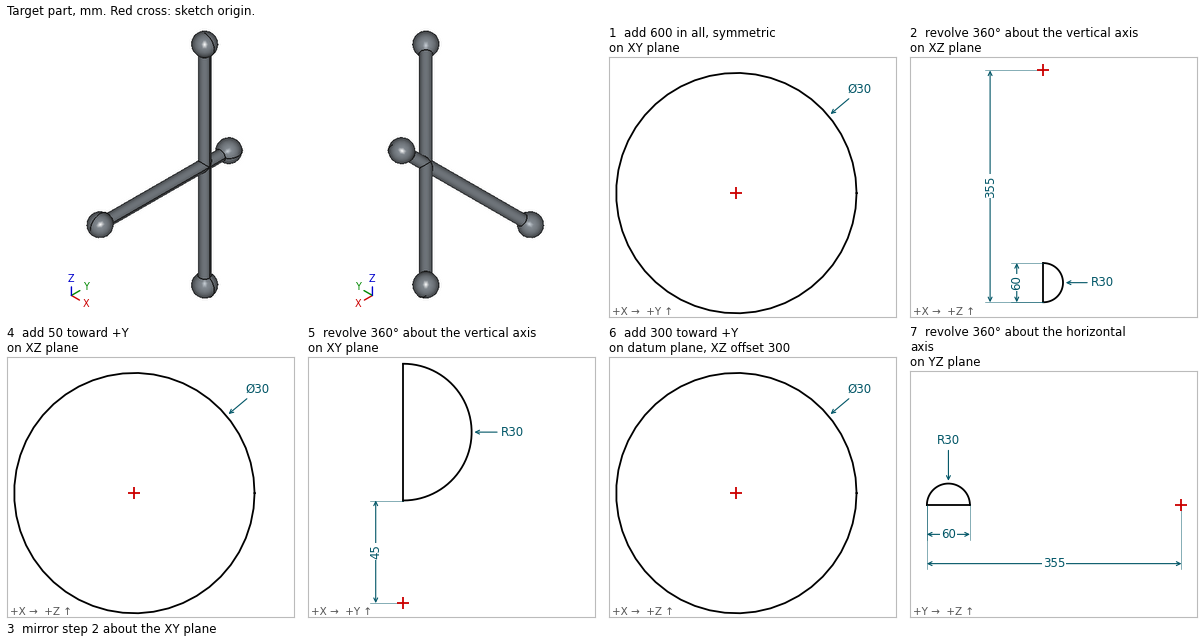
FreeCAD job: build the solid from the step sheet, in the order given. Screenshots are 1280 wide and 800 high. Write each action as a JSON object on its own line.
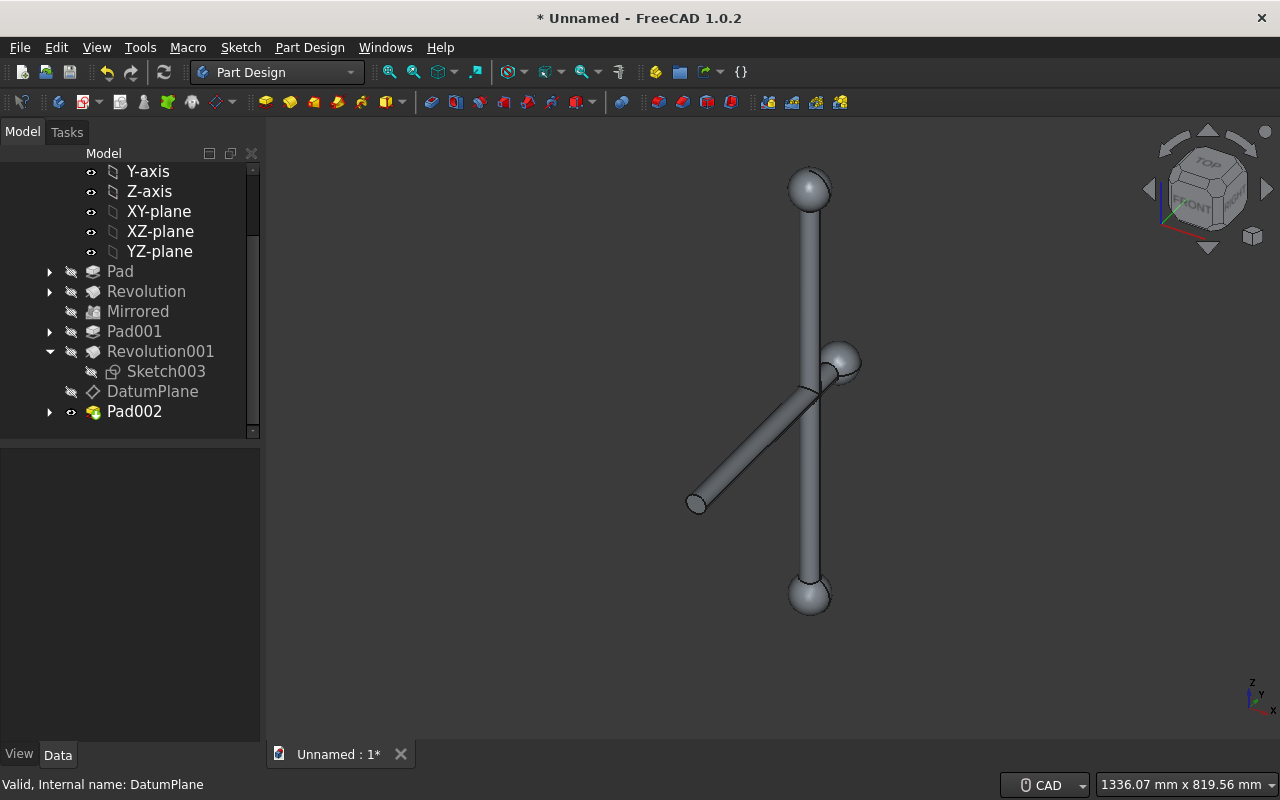
{"action": "left_click", "coordinate": [84, 102]}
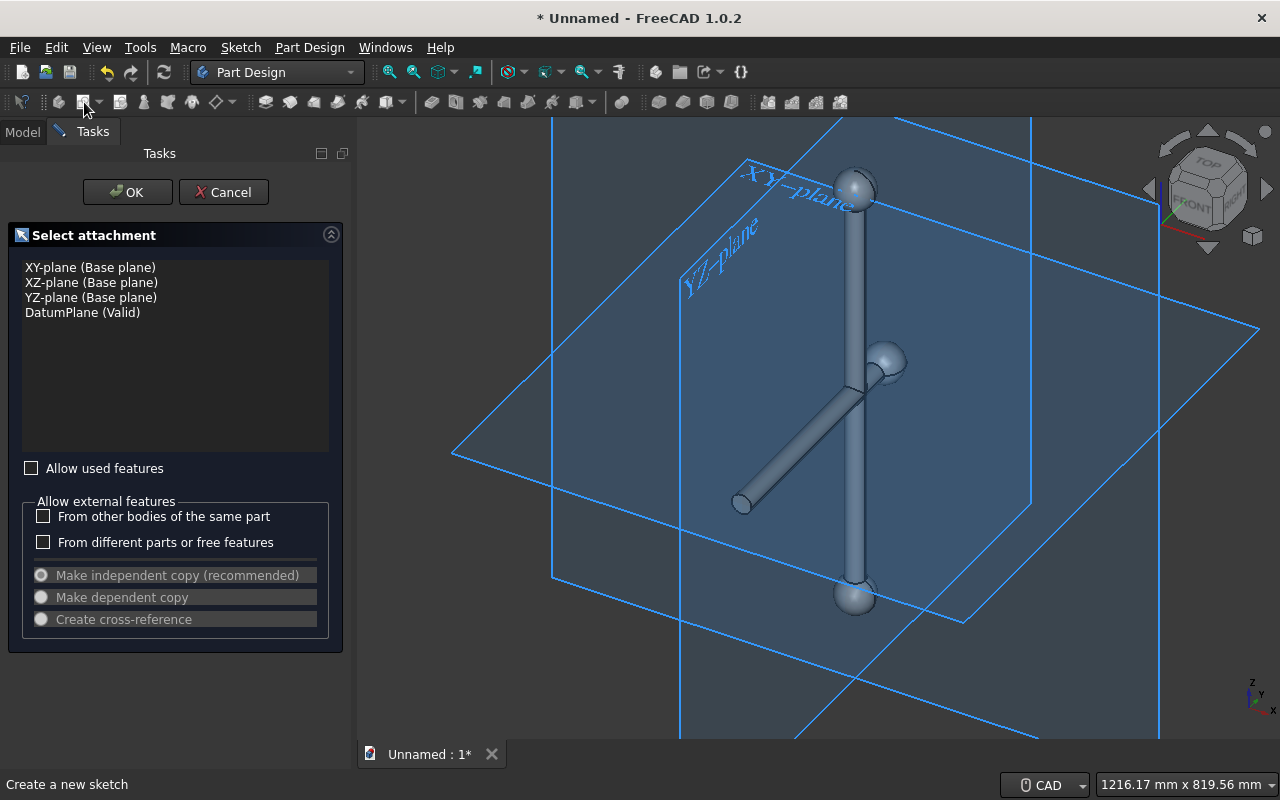
{"action": "left_click", "coordinate": [82, 298]}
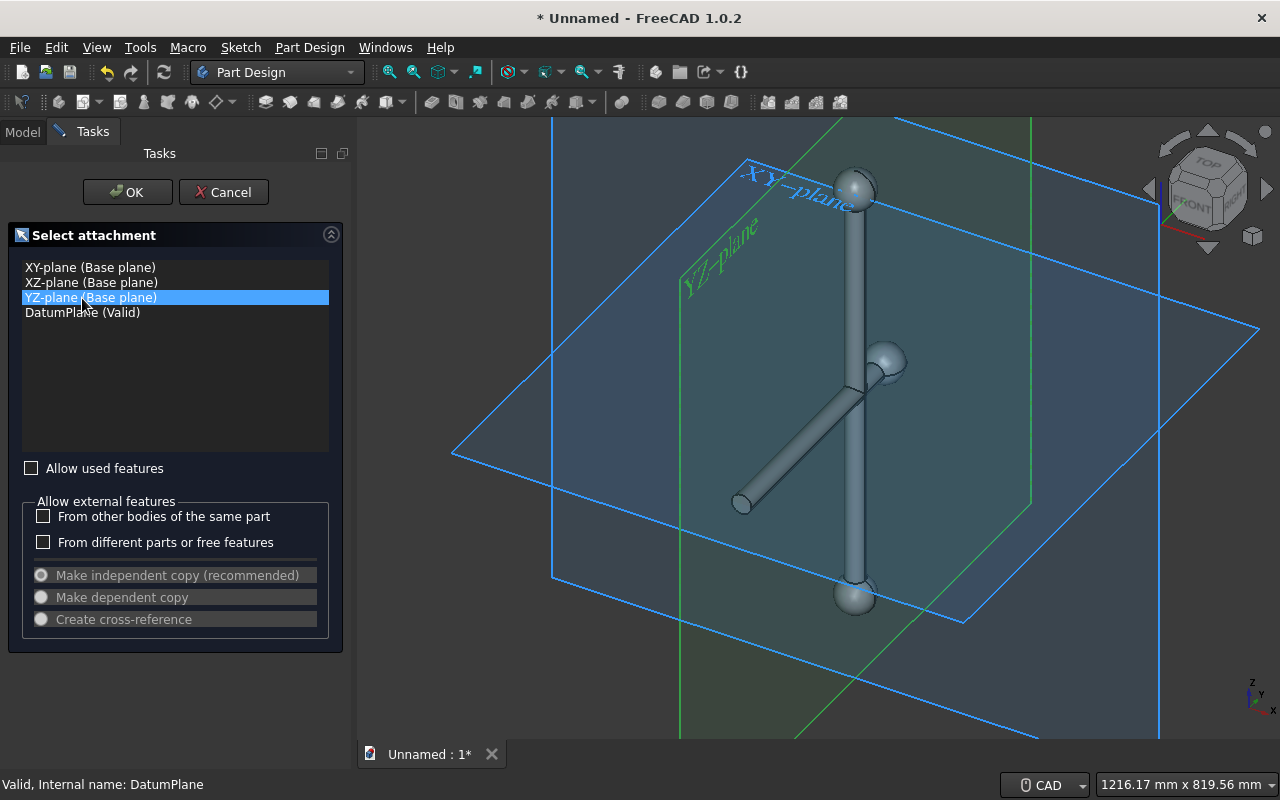
{"action": "left_click", "coordinate": [128, 192]}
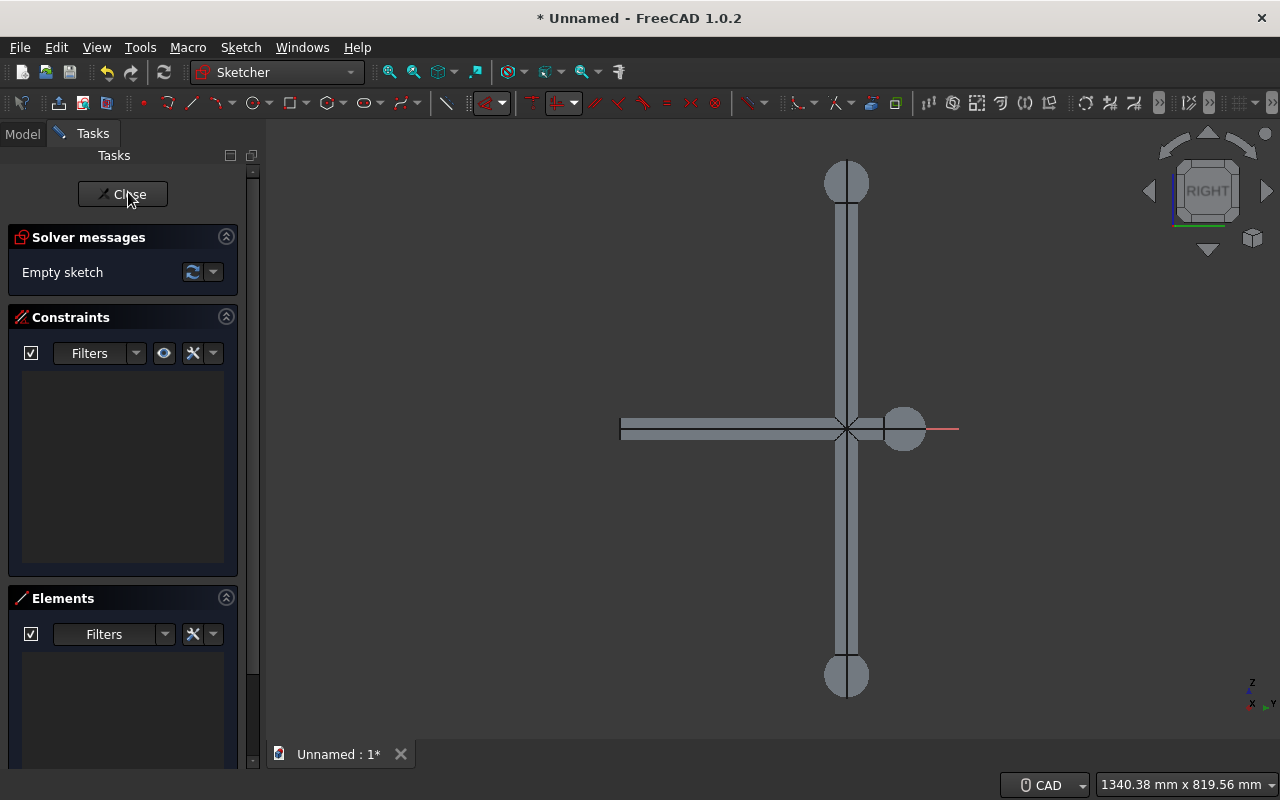
{"action": "key", "text": "q s"}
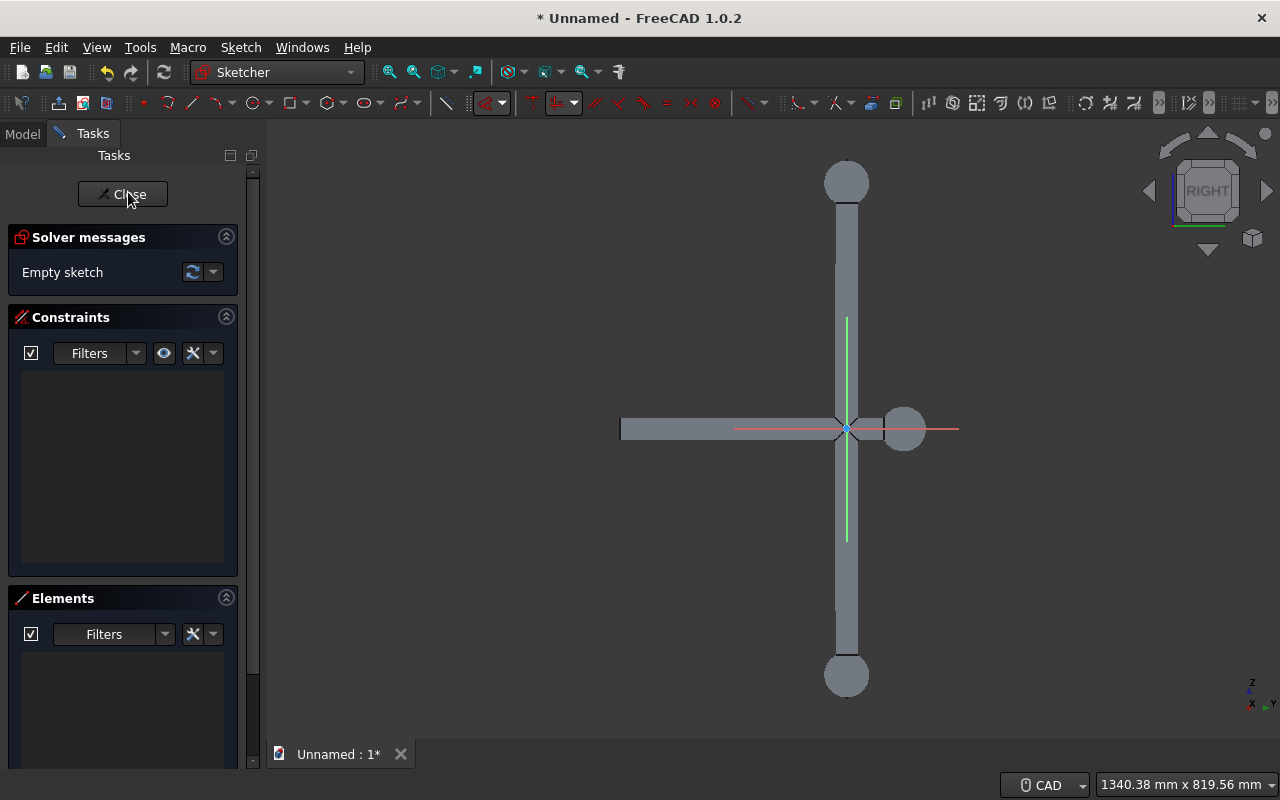
{"action": "scroll", "coordinate": [593, 417], "scroll_direction": "up", "scroll_amount": 13}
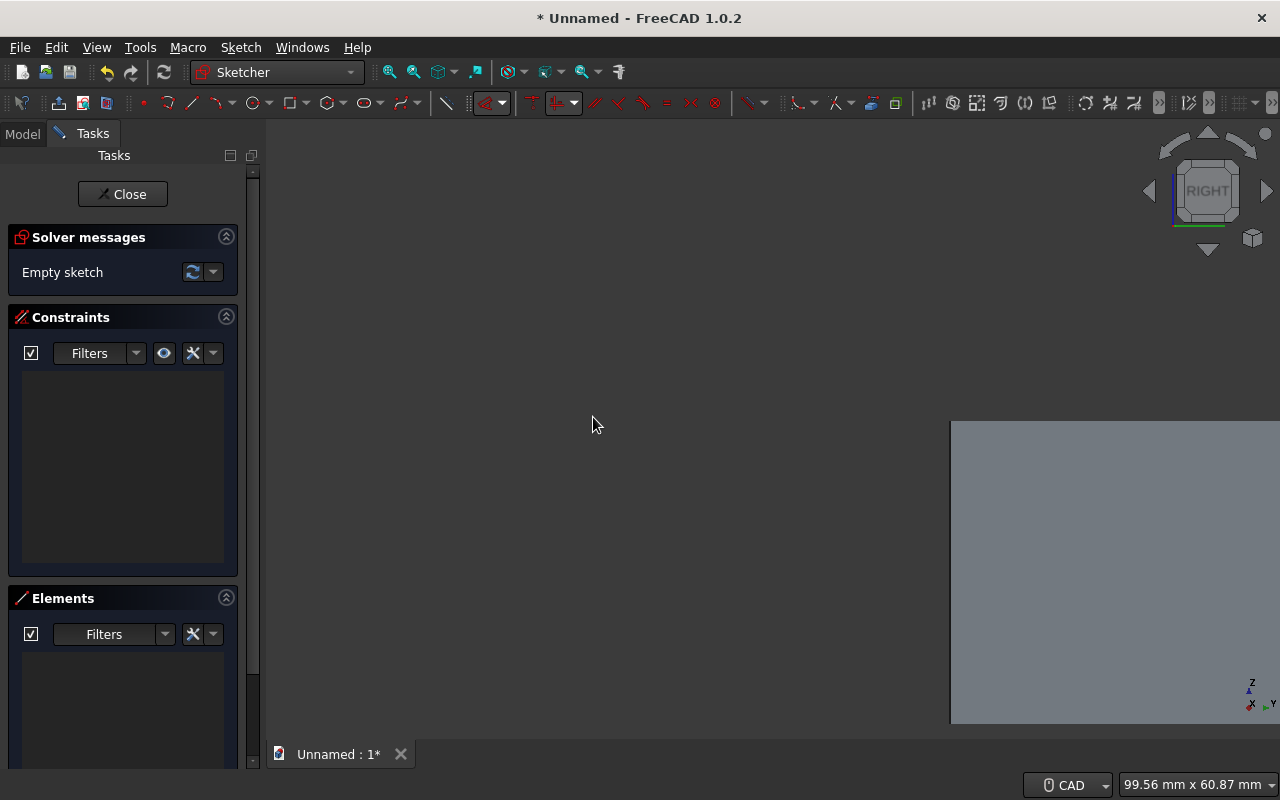
{"action": "left_click", "coordinate": [192, 104]}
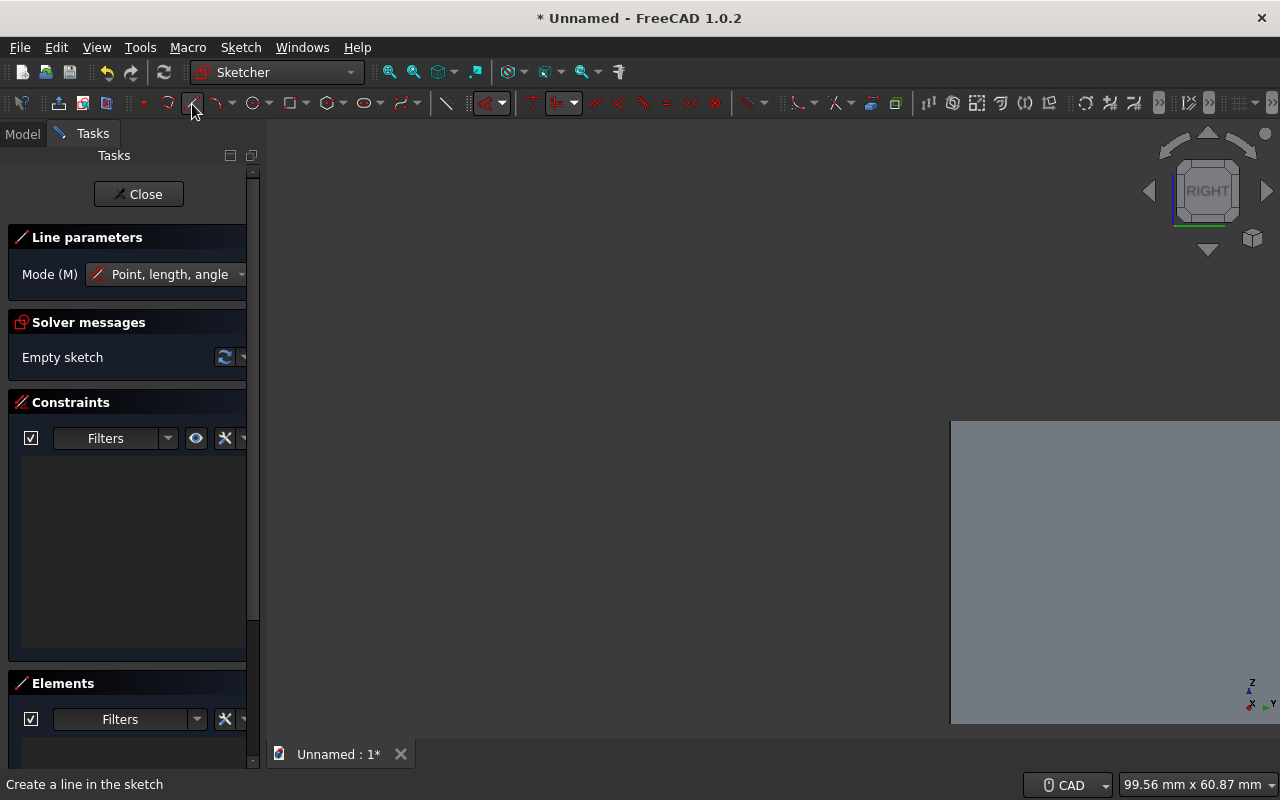
{"action": "left_click", "coordinate": [390, 573]}
{"action": "left_click", "coordinate": [1001, 564]}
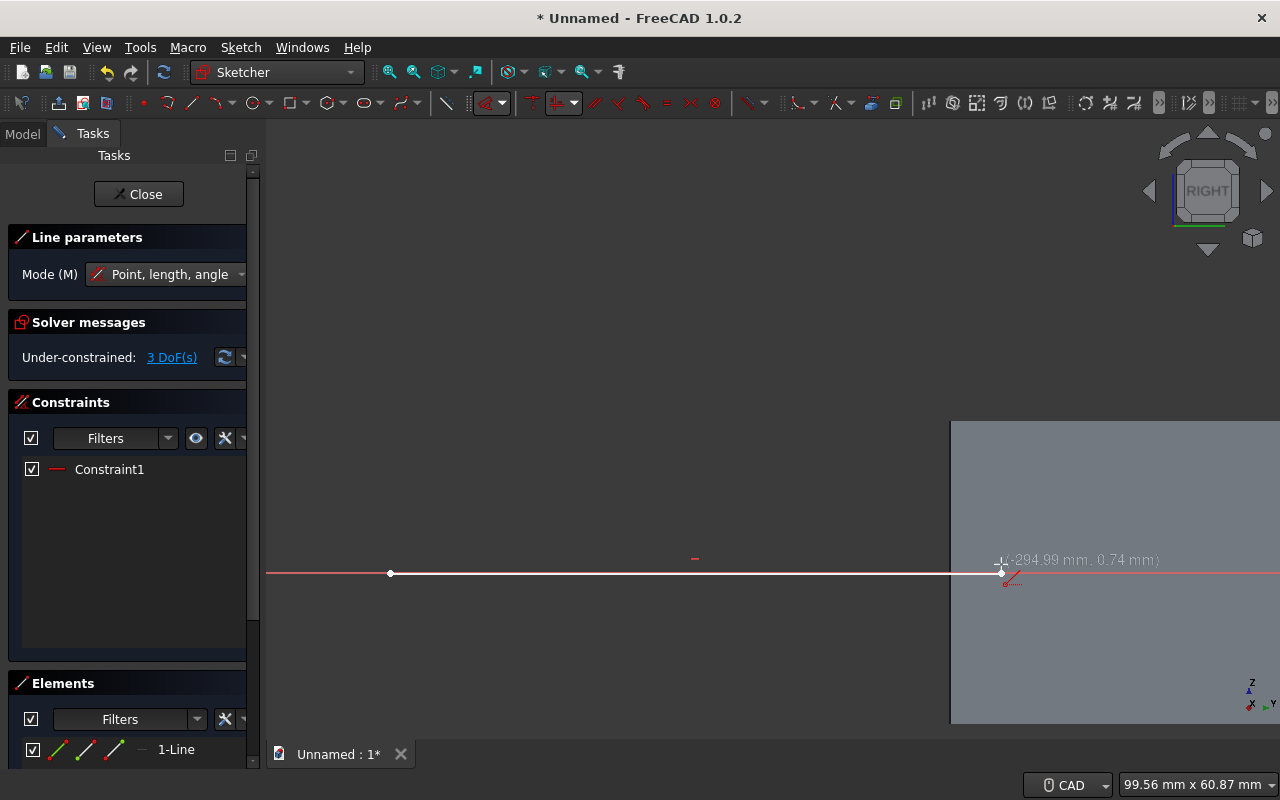
{"action": "left_click", "coordinate": [216, 104]}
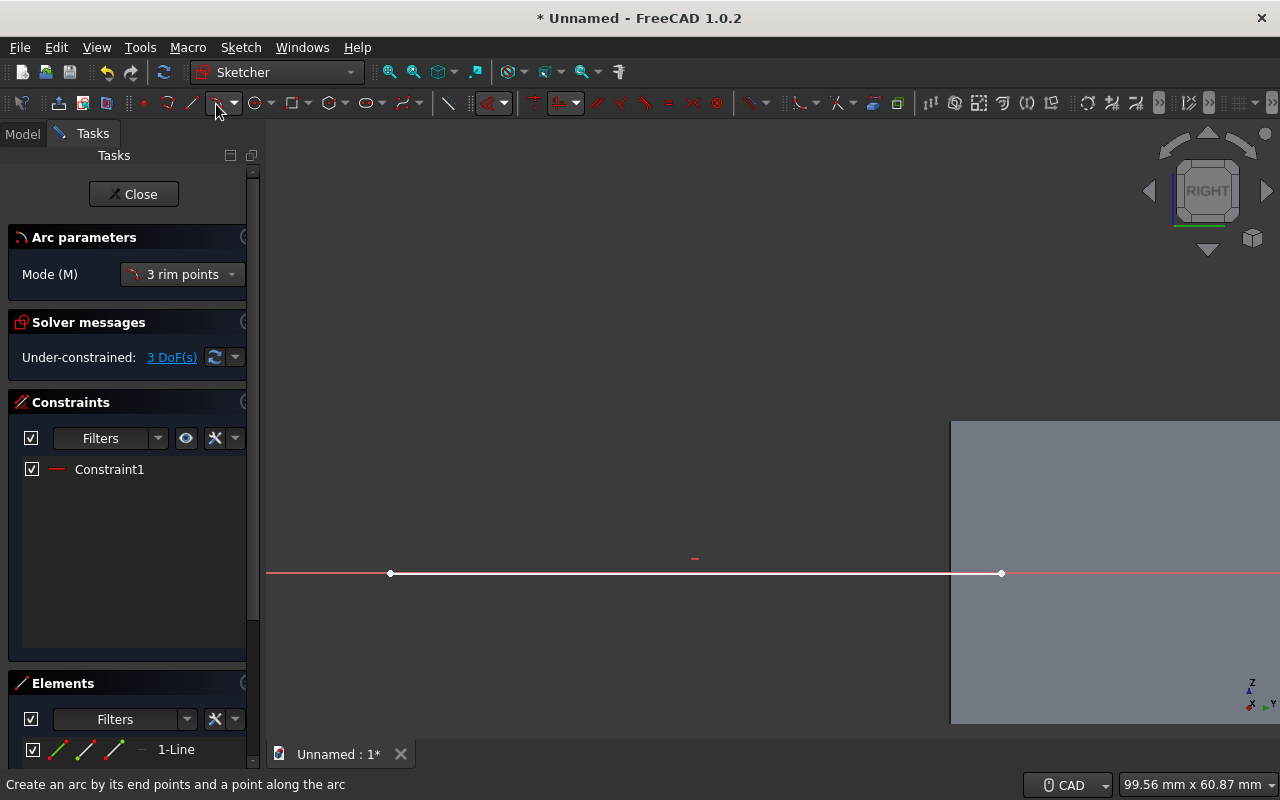
{"action": "left_click", "coordinate": [1001, 564]}
{"action": "left_click", "coordinate": [390, 574]}
{"action": "left_click", "coordinate": [695, 267]}
{"action": "key", "text": "Escape"}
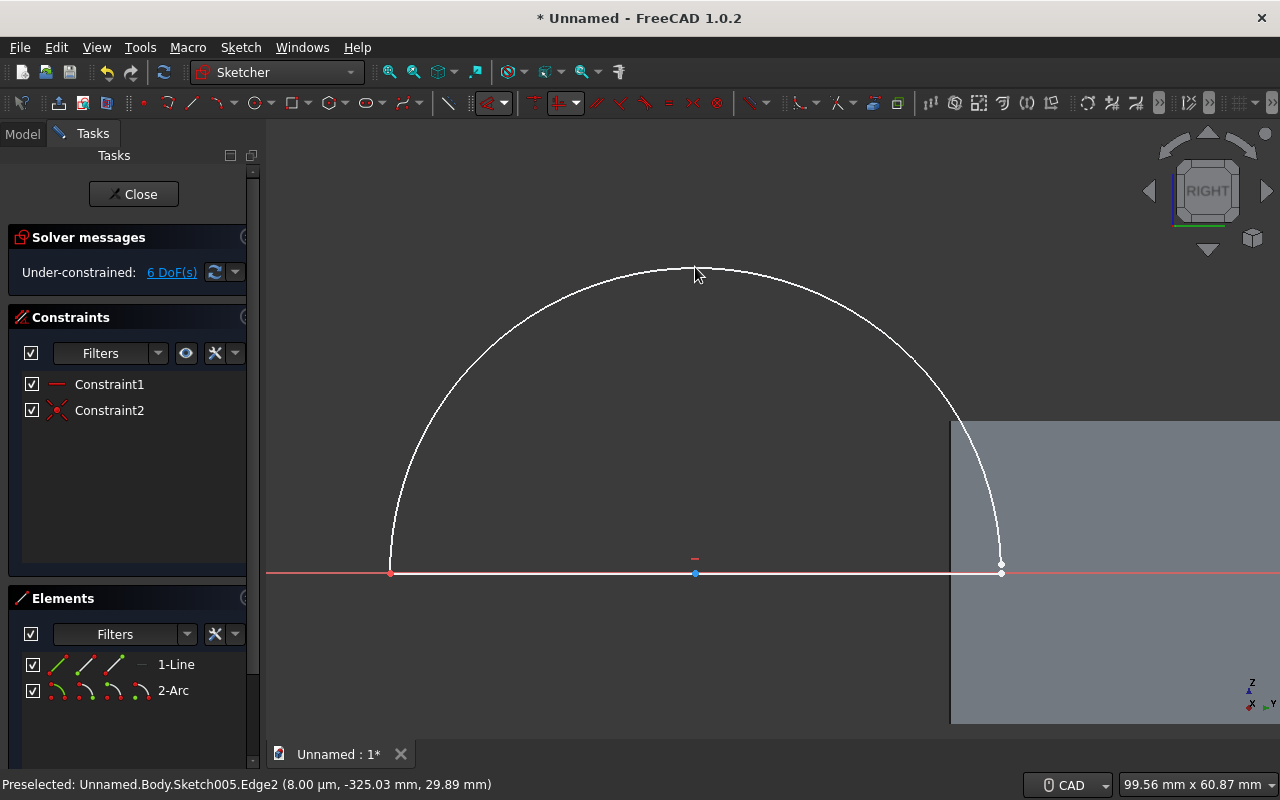
{"action": "left_click", "coordinate": [696, 574]}